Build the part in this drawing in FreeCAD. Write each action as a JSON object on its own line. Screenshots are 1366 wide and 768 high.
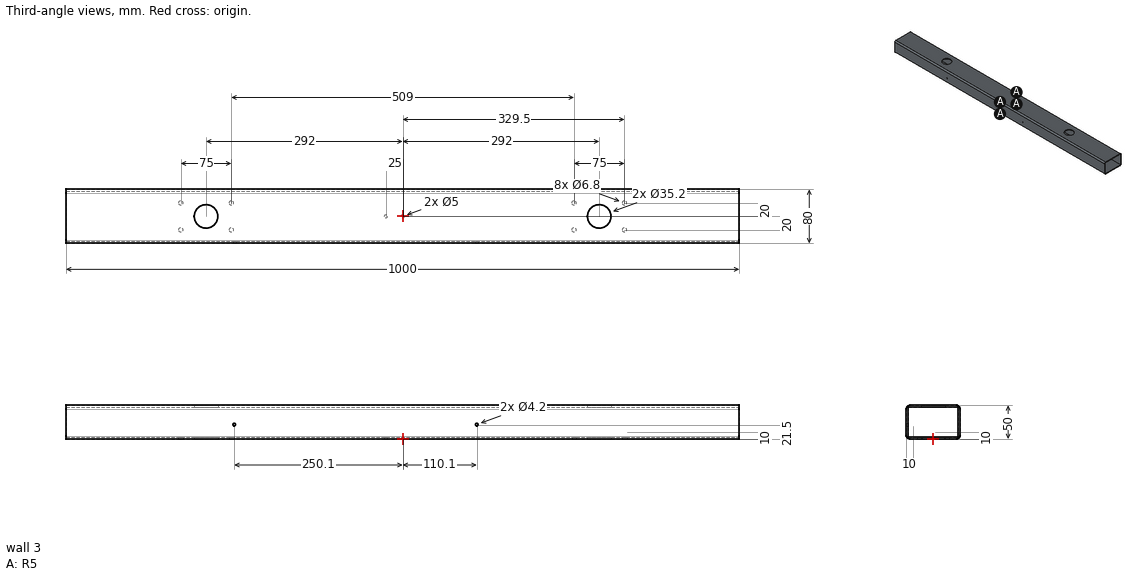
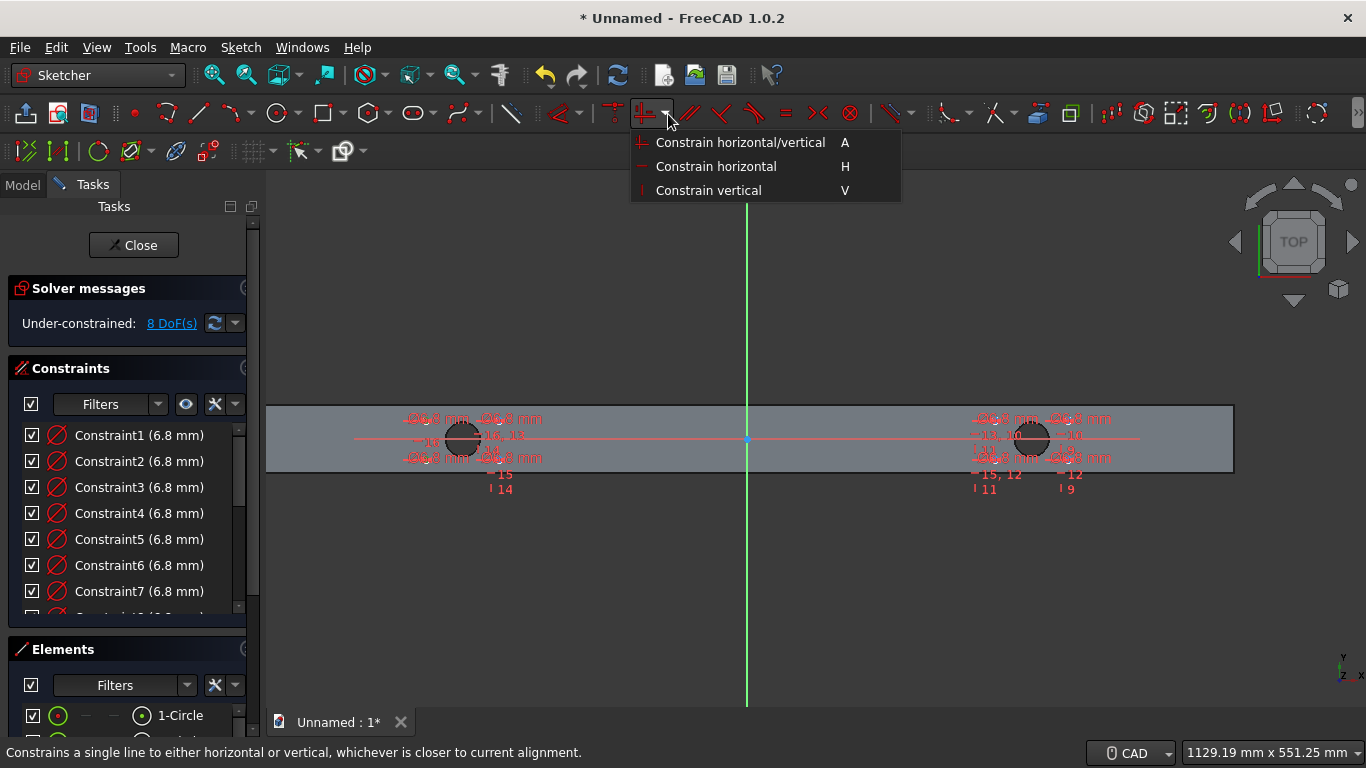
{"action": "left_click", "coordinate": [766, 190]}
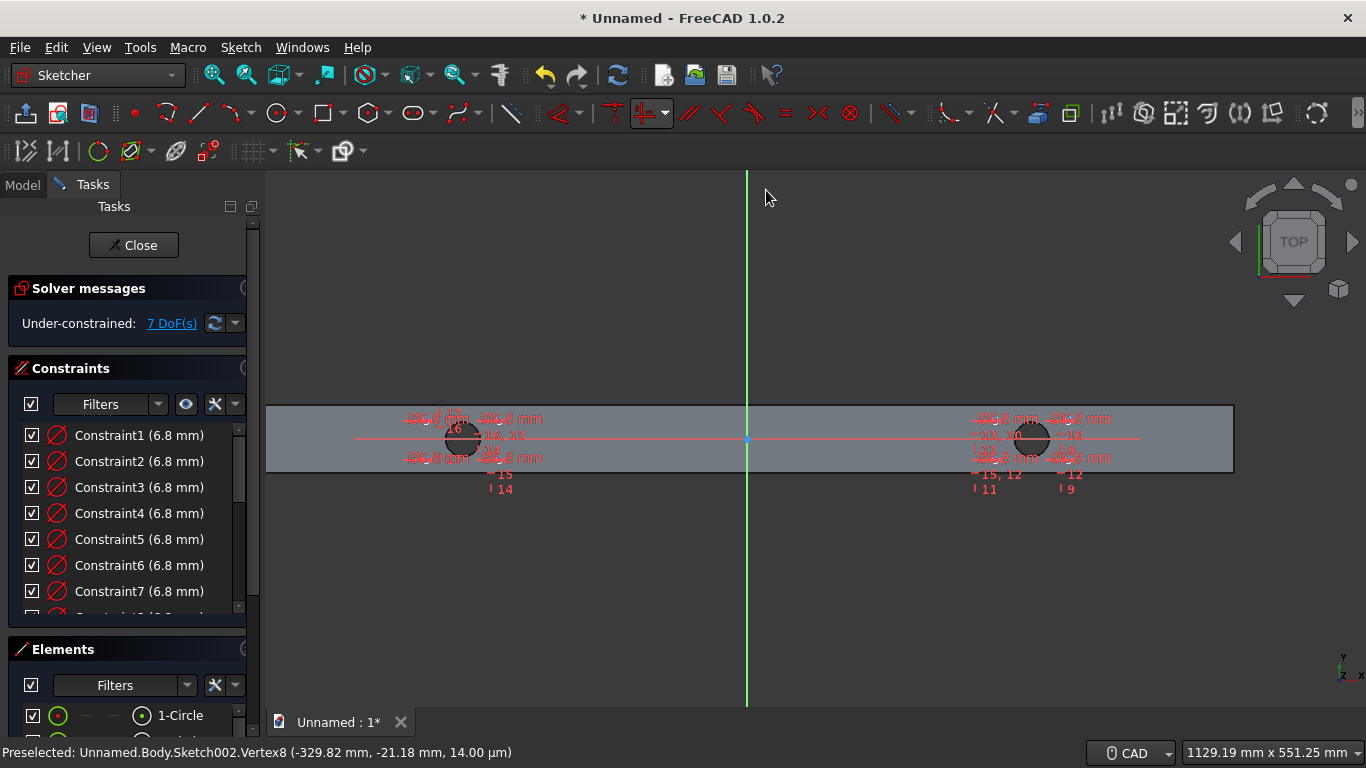
{"action": "left_click", "coordinate": [499, 460]}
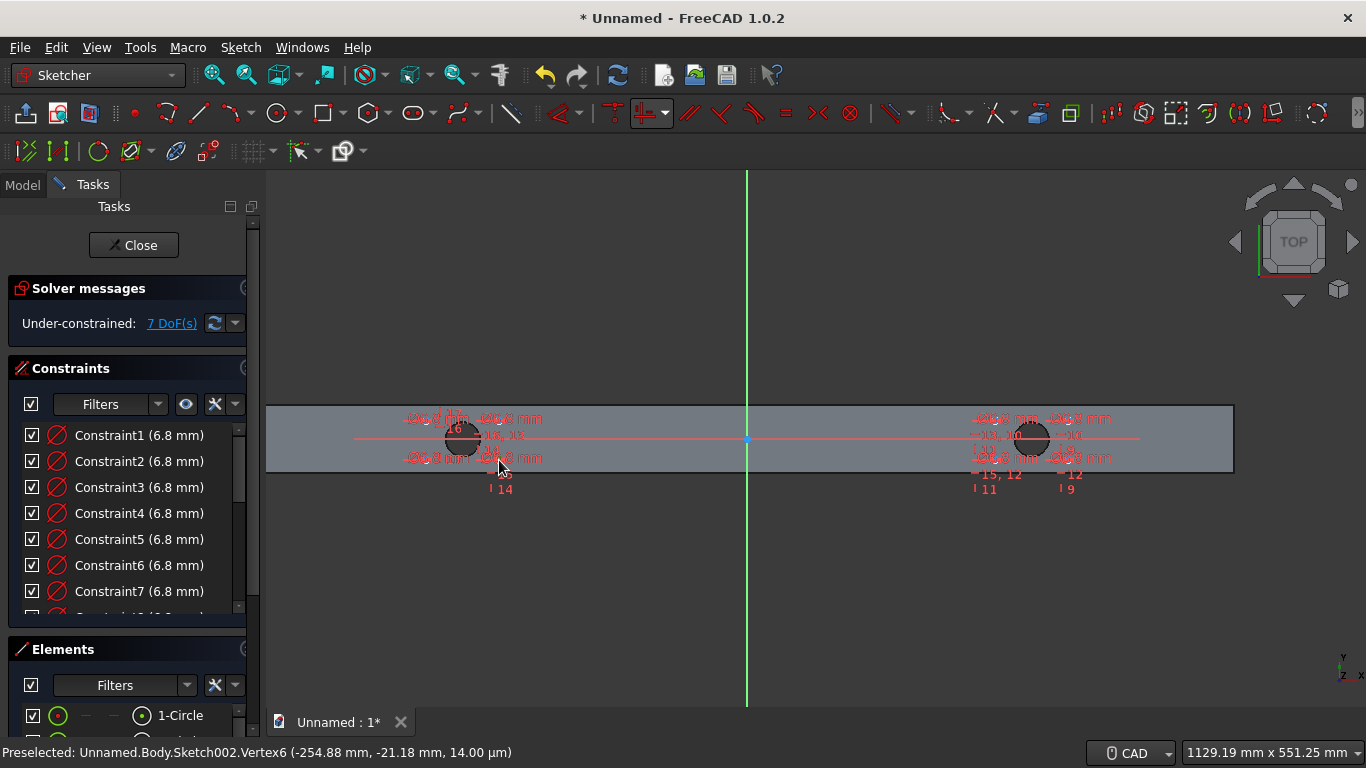
{"action": "left_click", "coordinate": [426, 460]}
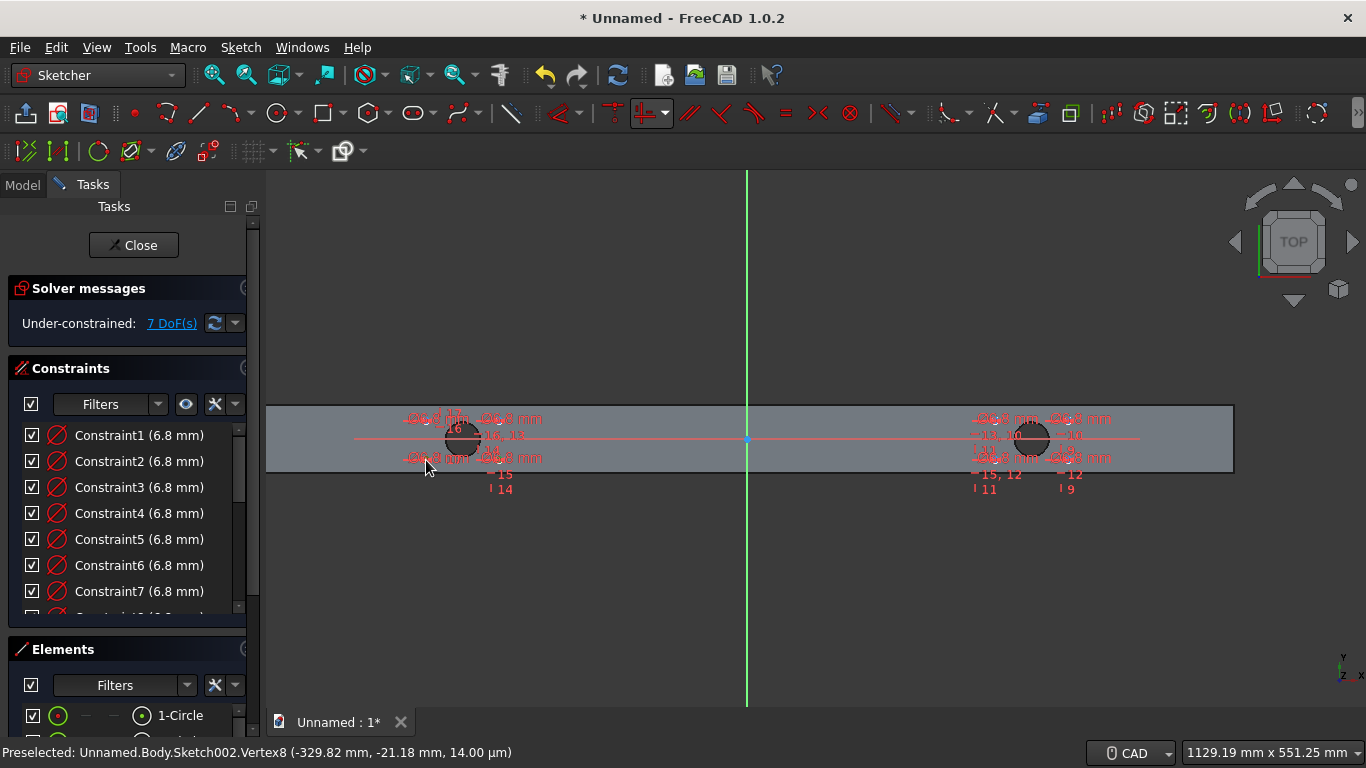
{"action": "key", "text": "h"}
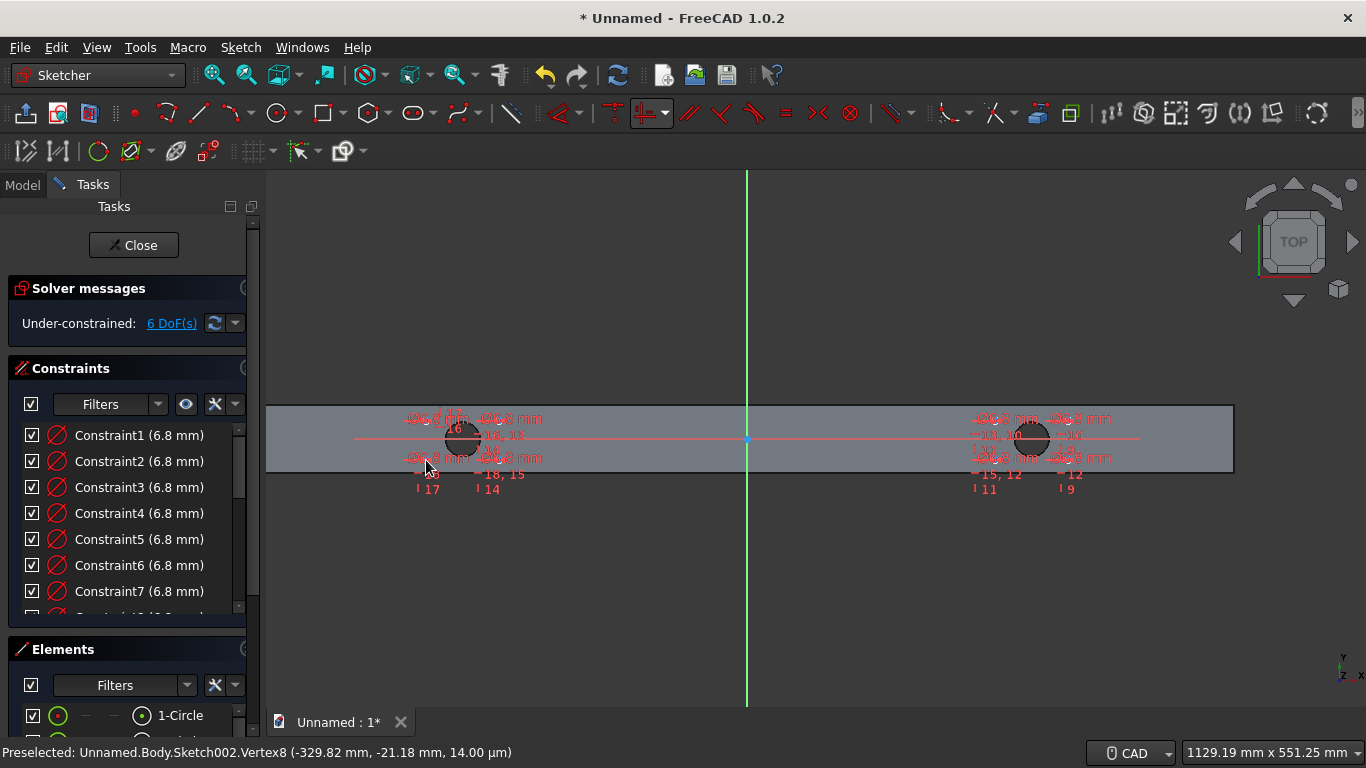
{"action": "scroll", "coordinate": [1068, 421], "scroll_direction": "up", "scroll_amount": 4}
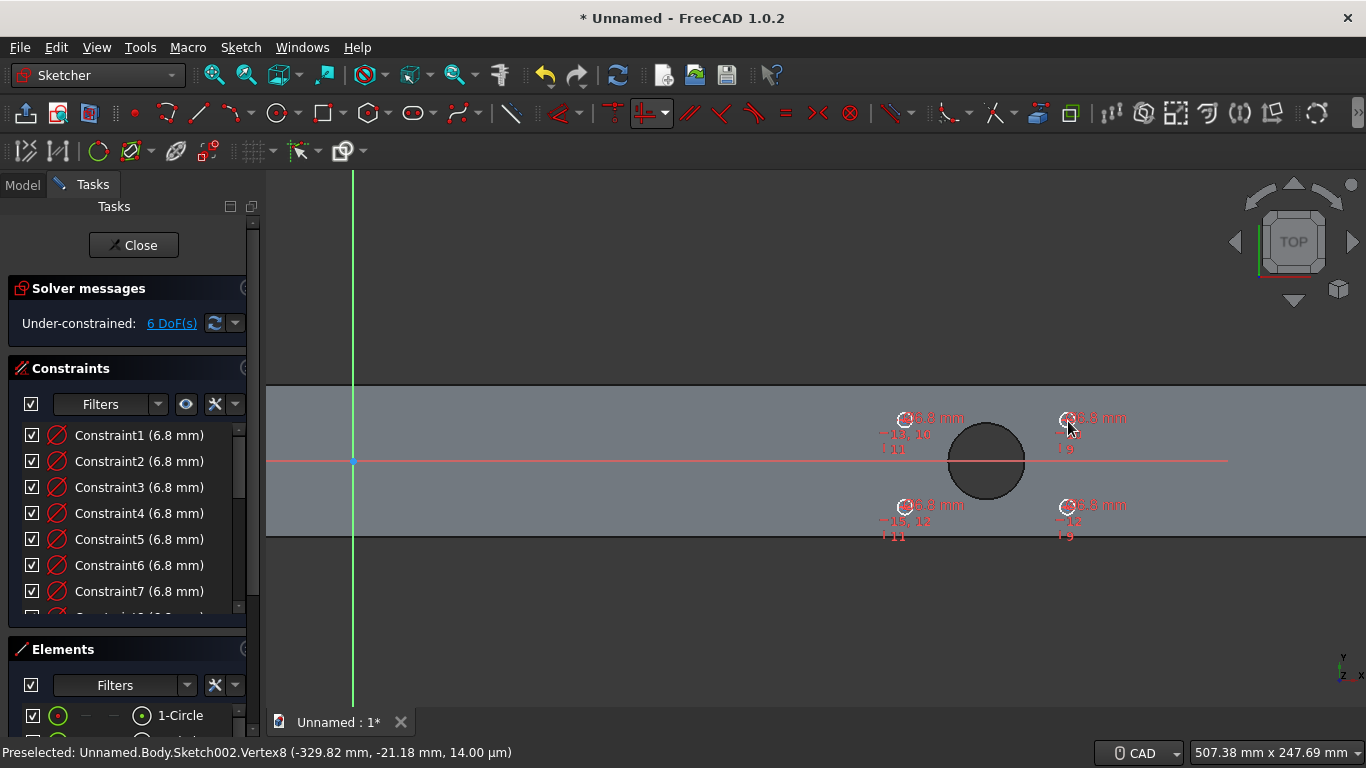
{"action": "left_click", "coordinate": [1067, 420]}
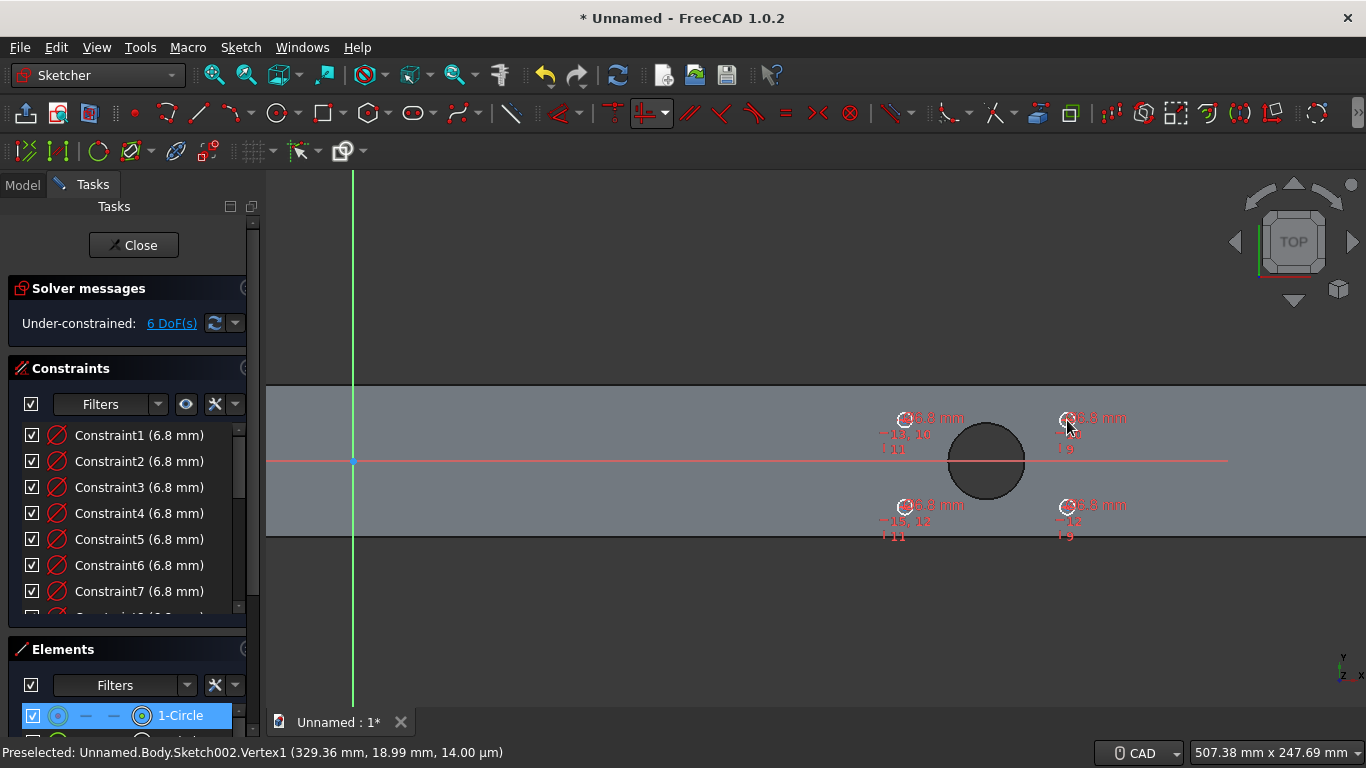
{"action": "left_click", "coordinate": [582, 114]}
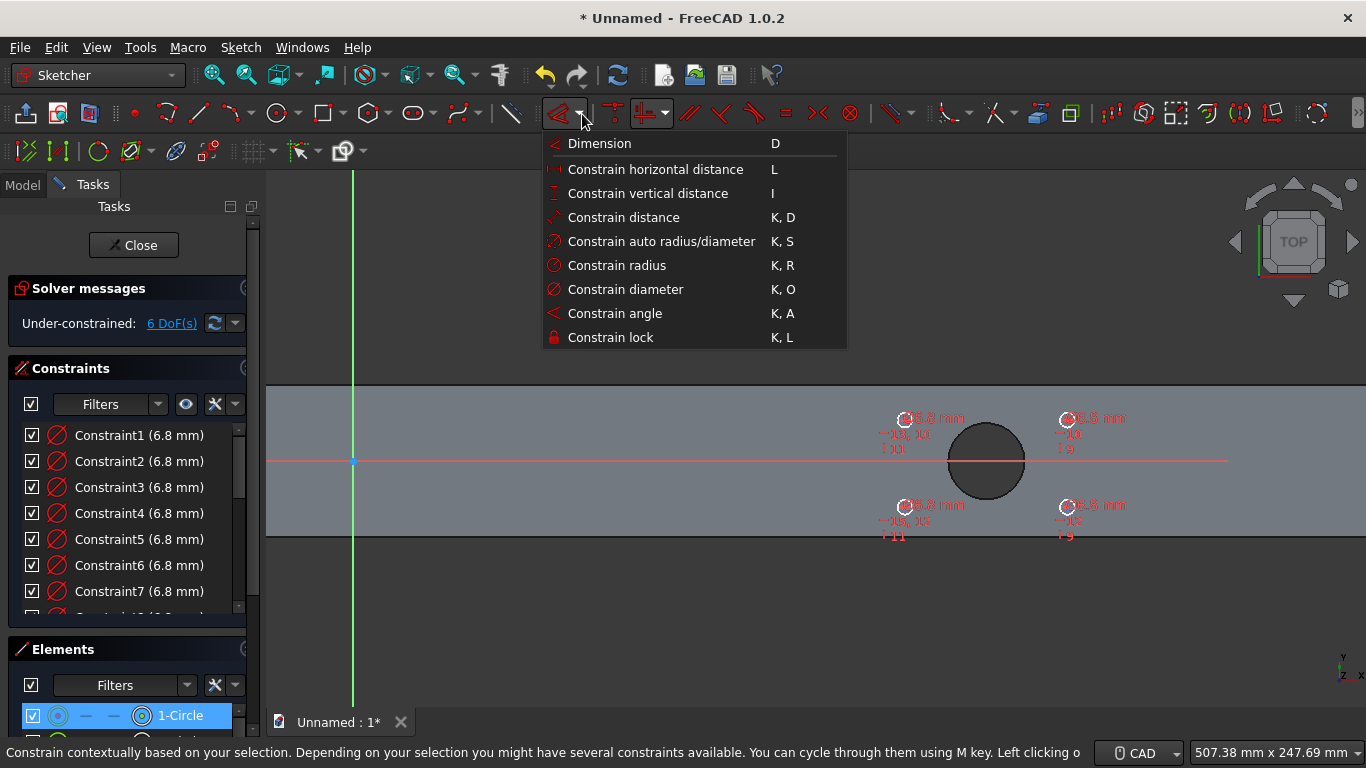
{"action": "left_click", "coordinate": [695, 193]}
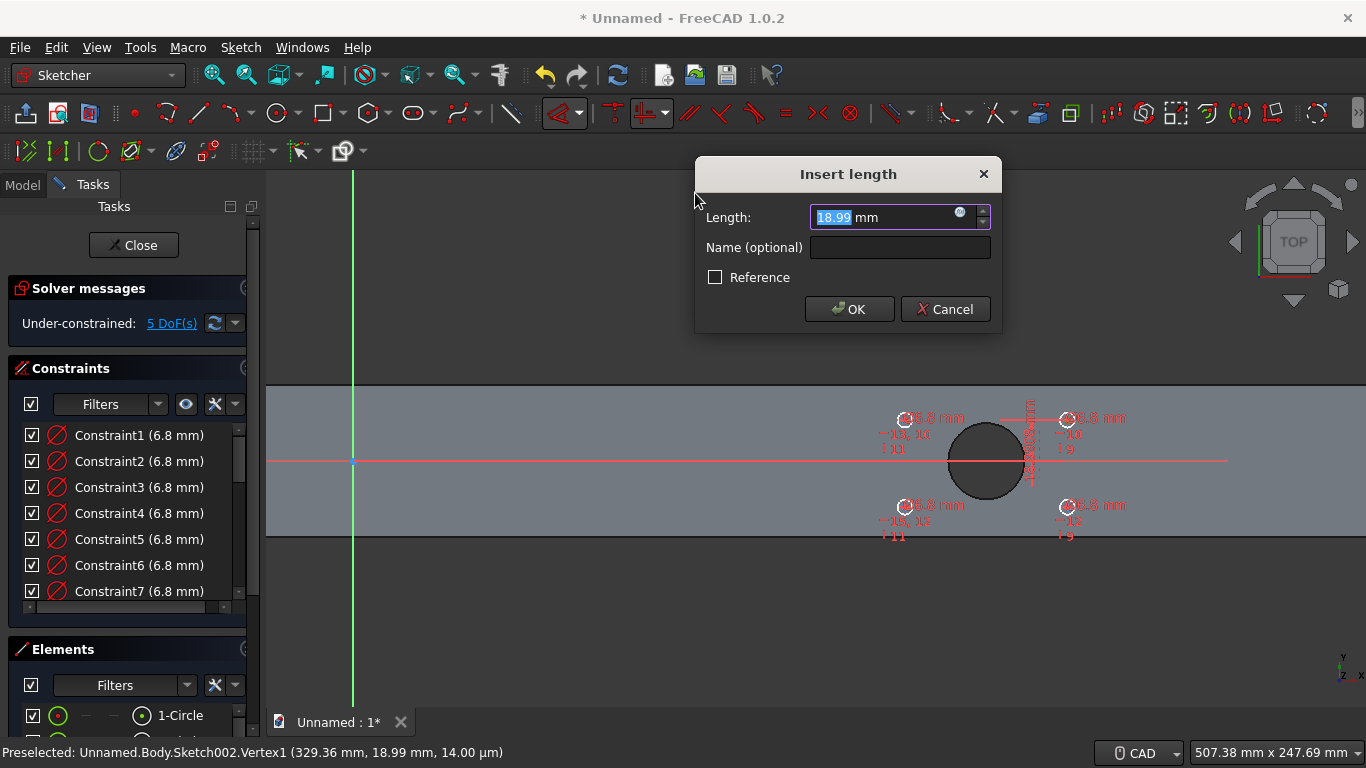
{"action": "type", "text": "20"}
{"action": "key", "text": "Return"}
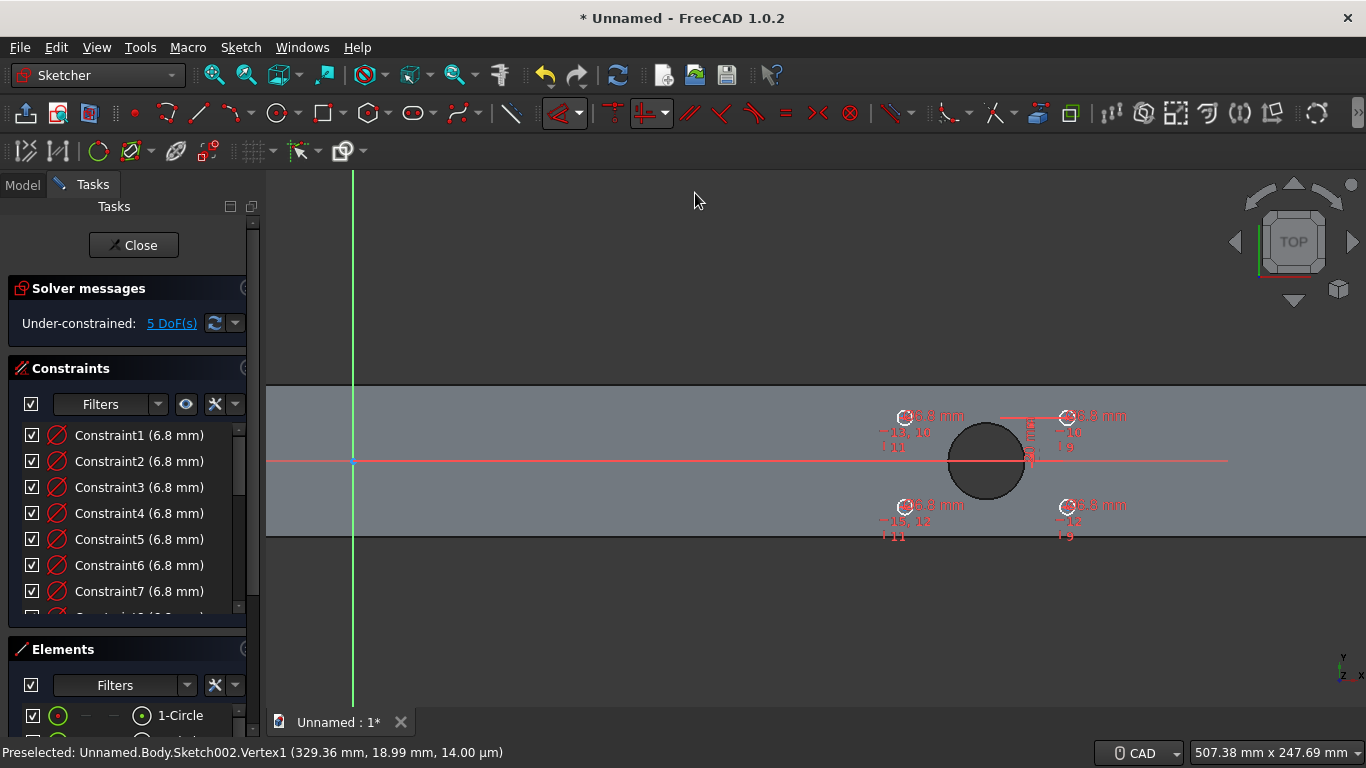
{"action": "left_click", "coordinate": [1067, 507]}